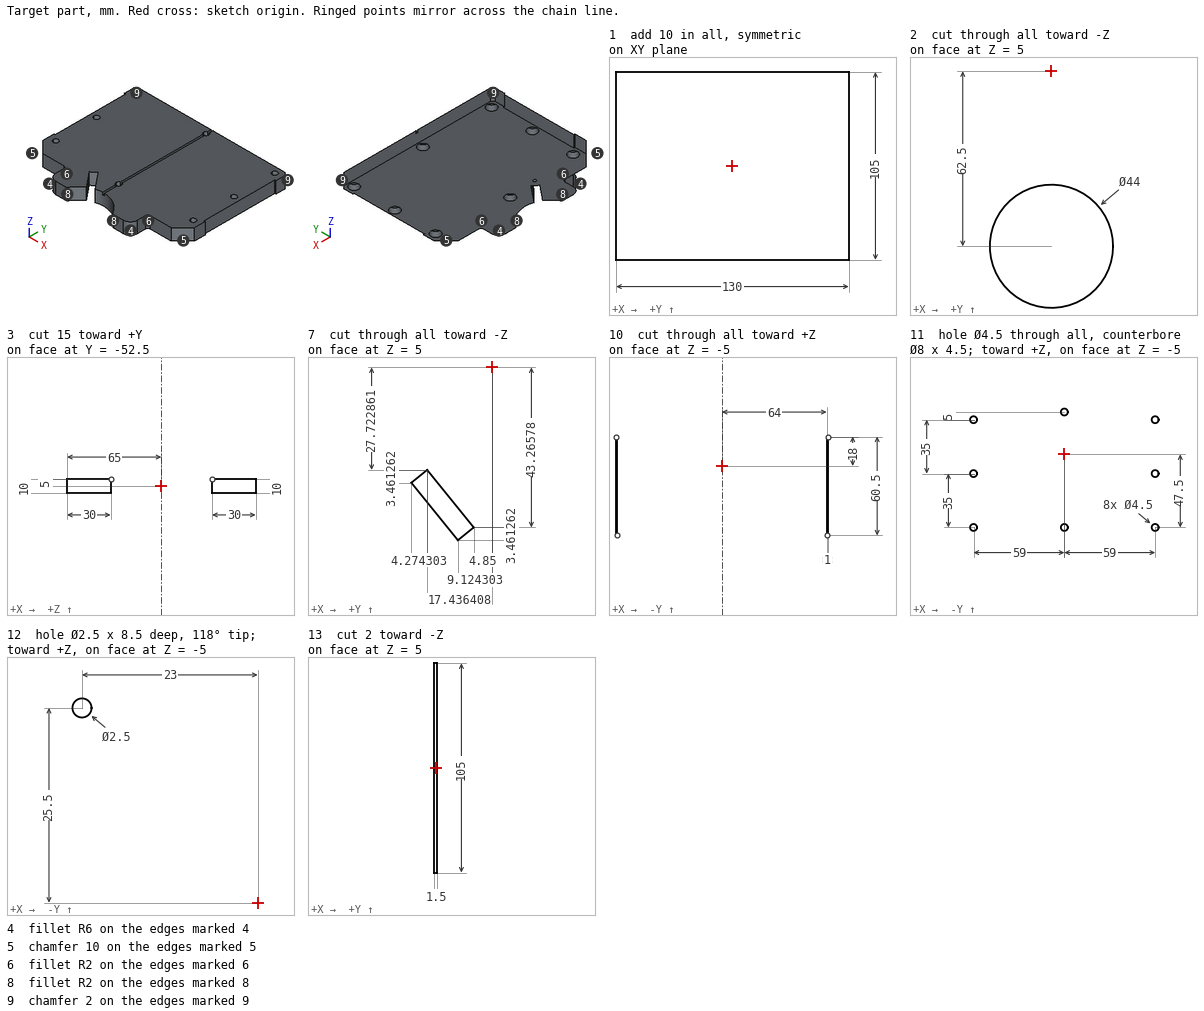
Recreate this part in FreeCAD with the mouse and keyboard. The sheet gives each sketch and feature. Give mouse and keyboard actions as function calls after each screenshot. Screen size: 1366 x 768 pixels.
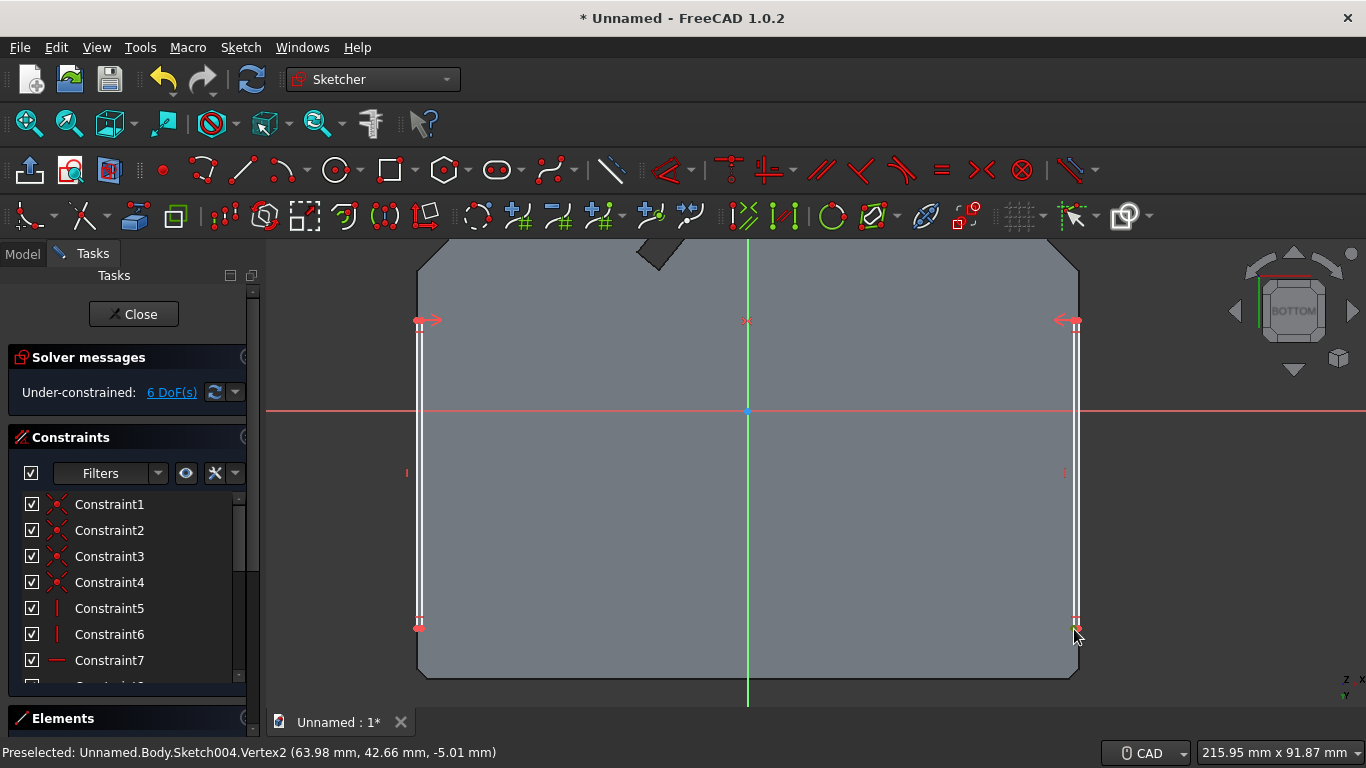
scroll(422, 629, up, 5)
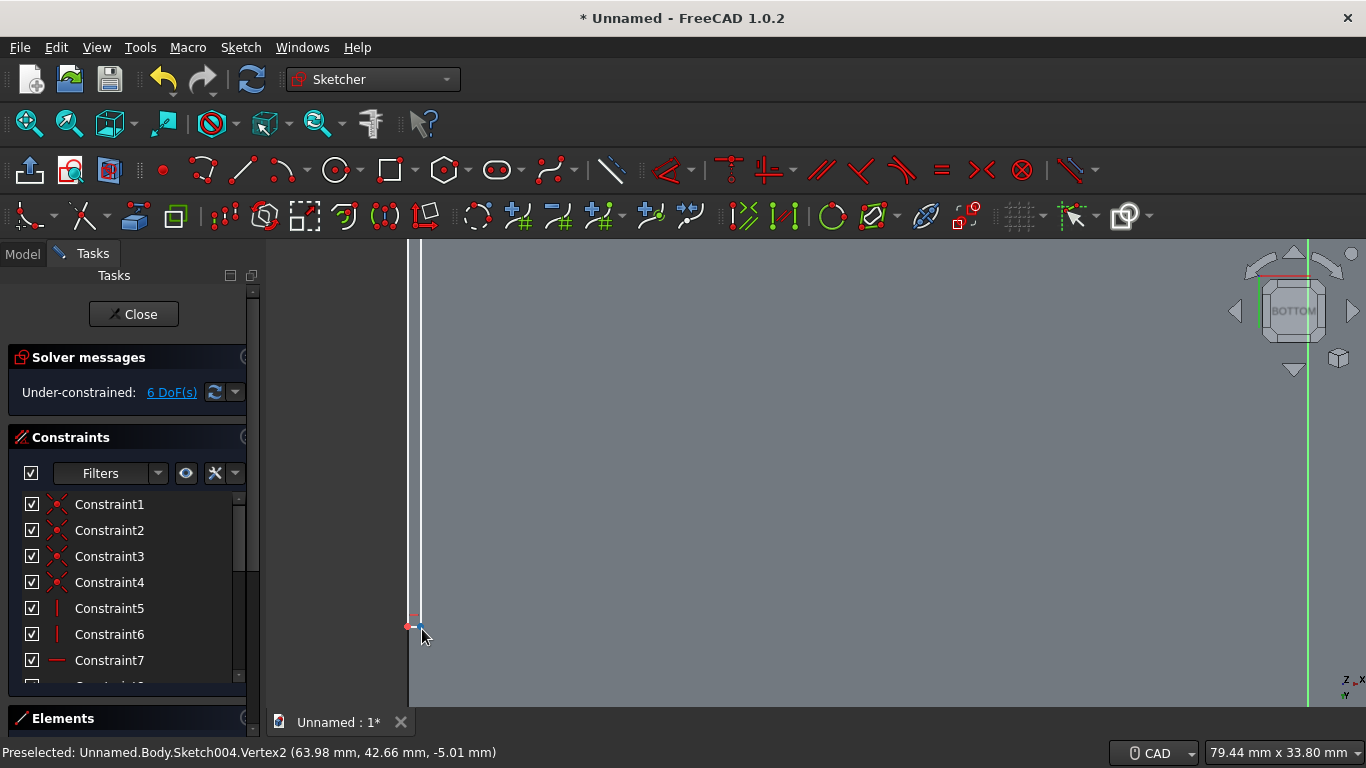
click(421, 627)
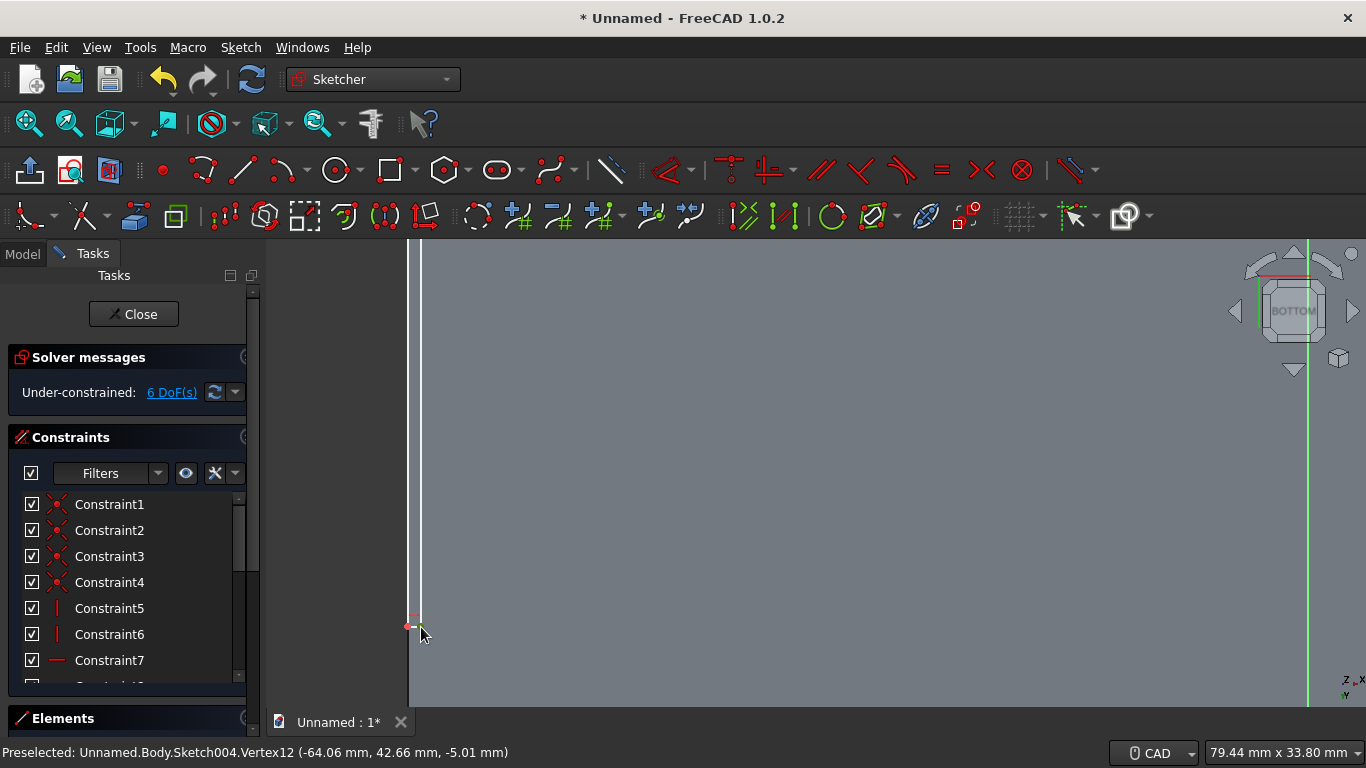
scroll(421, 629, down, 5)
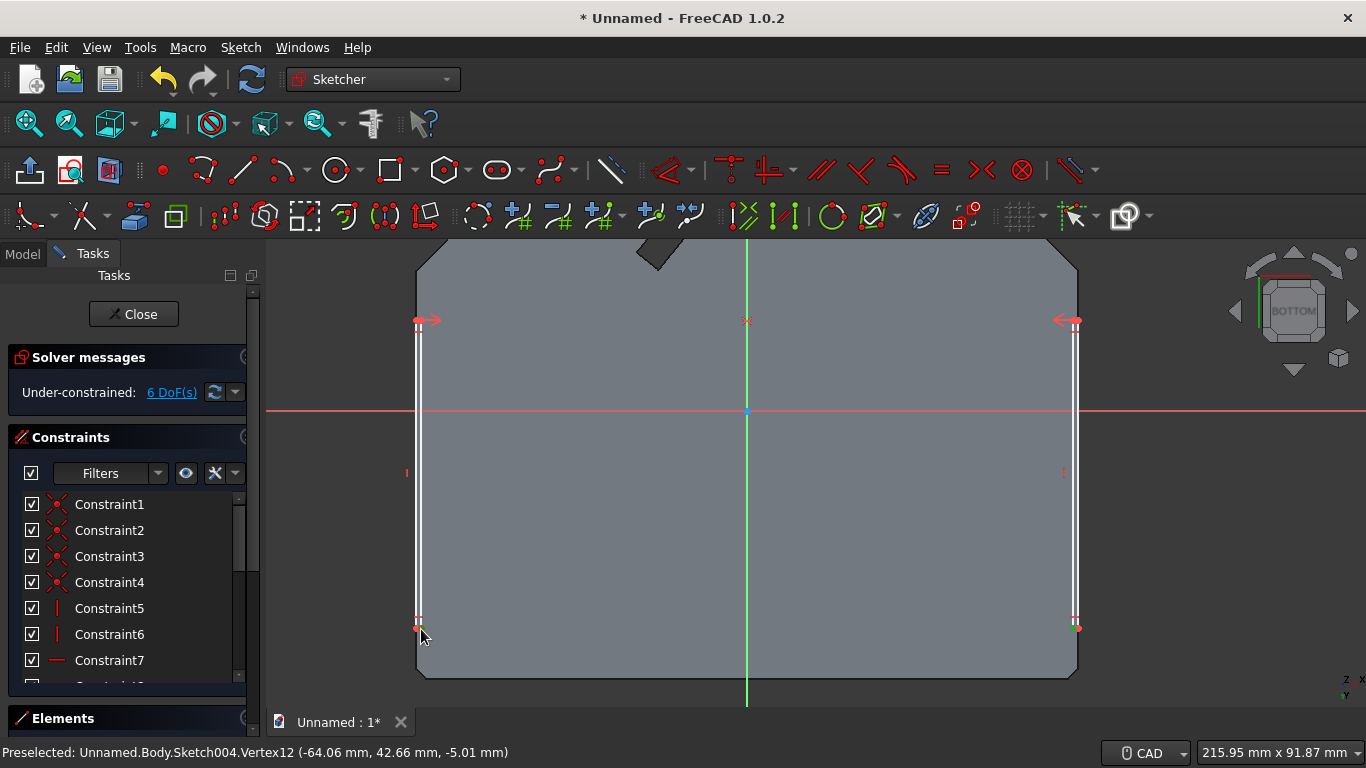
click(747, 650)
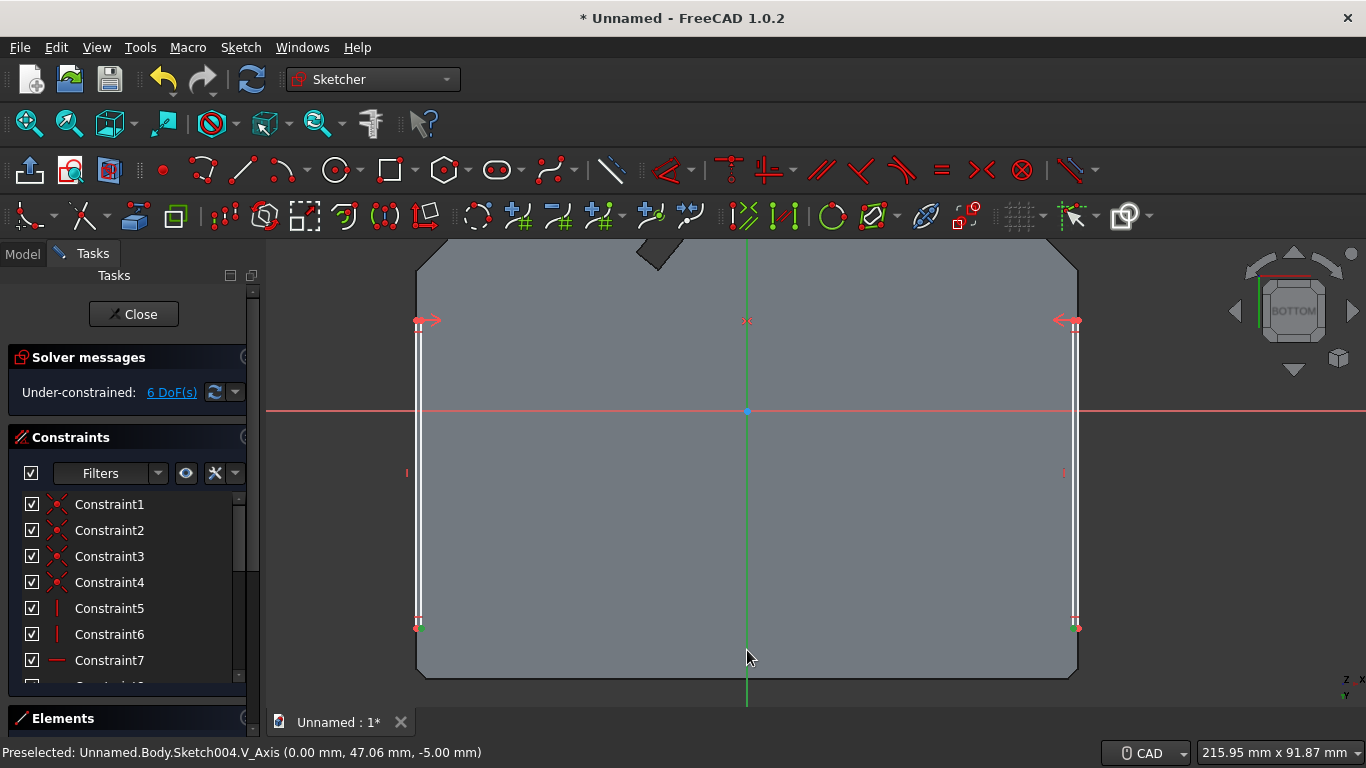
click(982, 170)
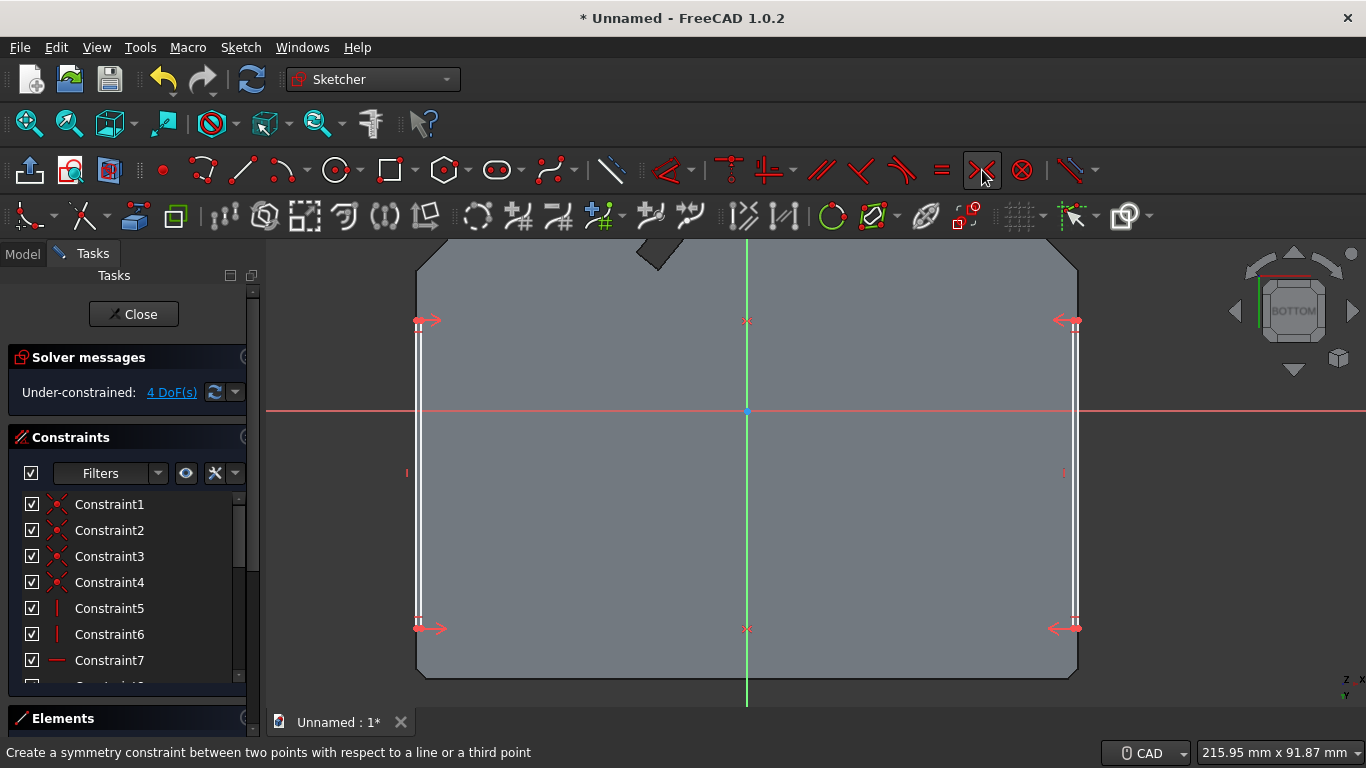
click(666, 170)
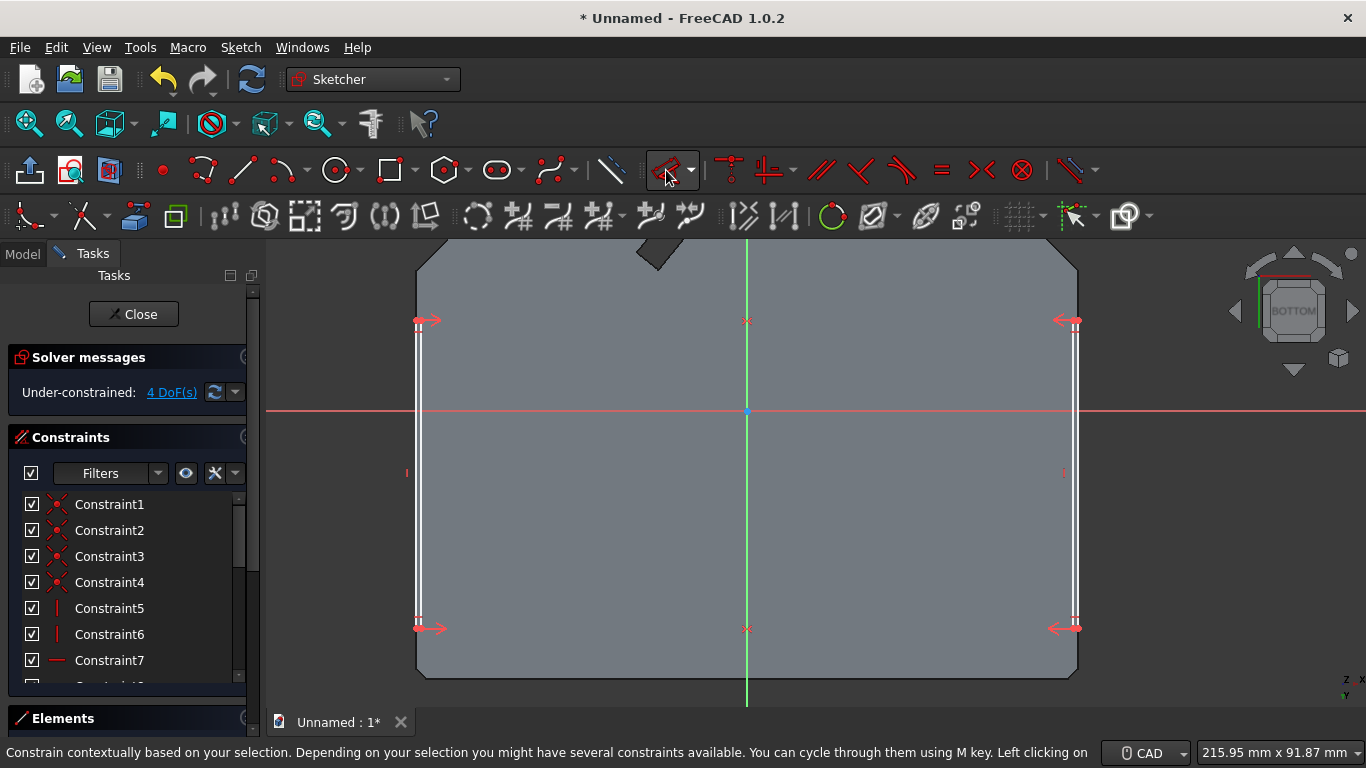
scroll(1076, 629, up, 11)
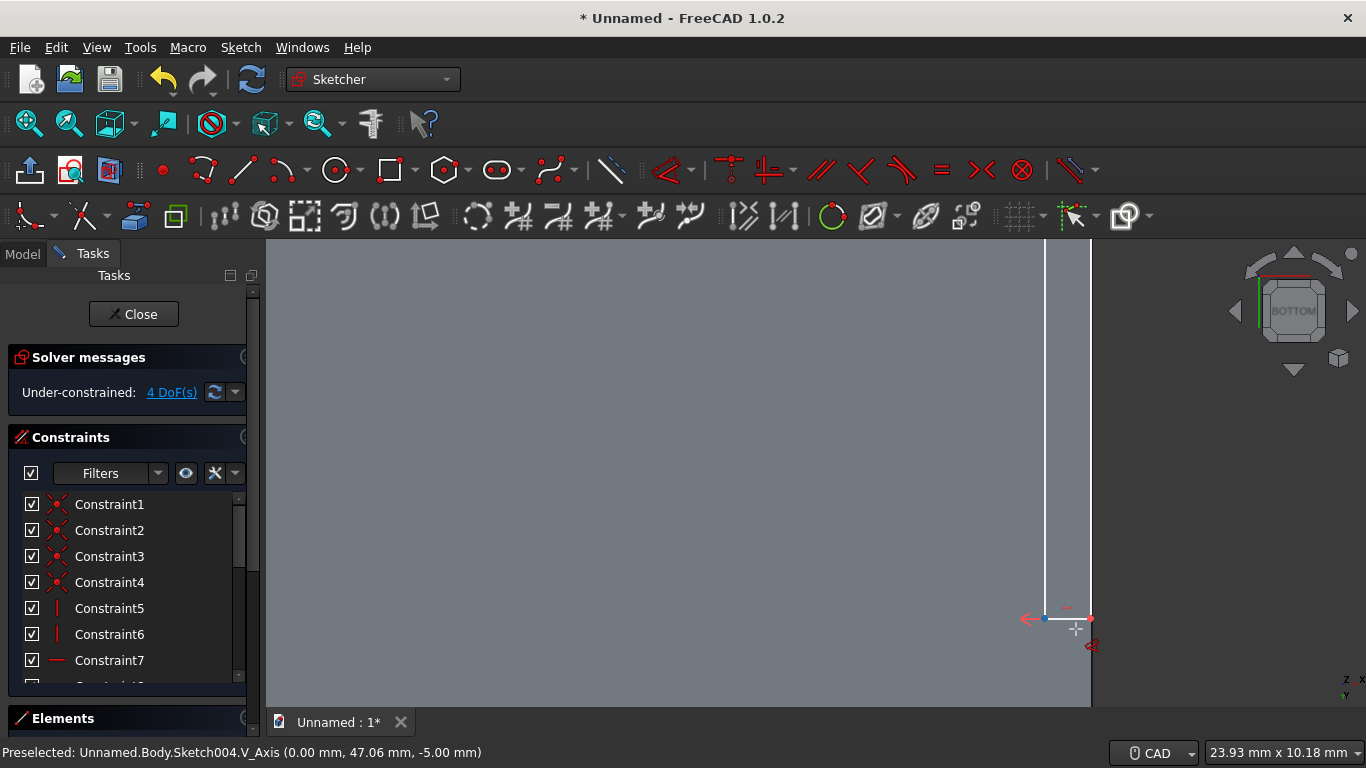
click(1068, 619)
click(1068, 653)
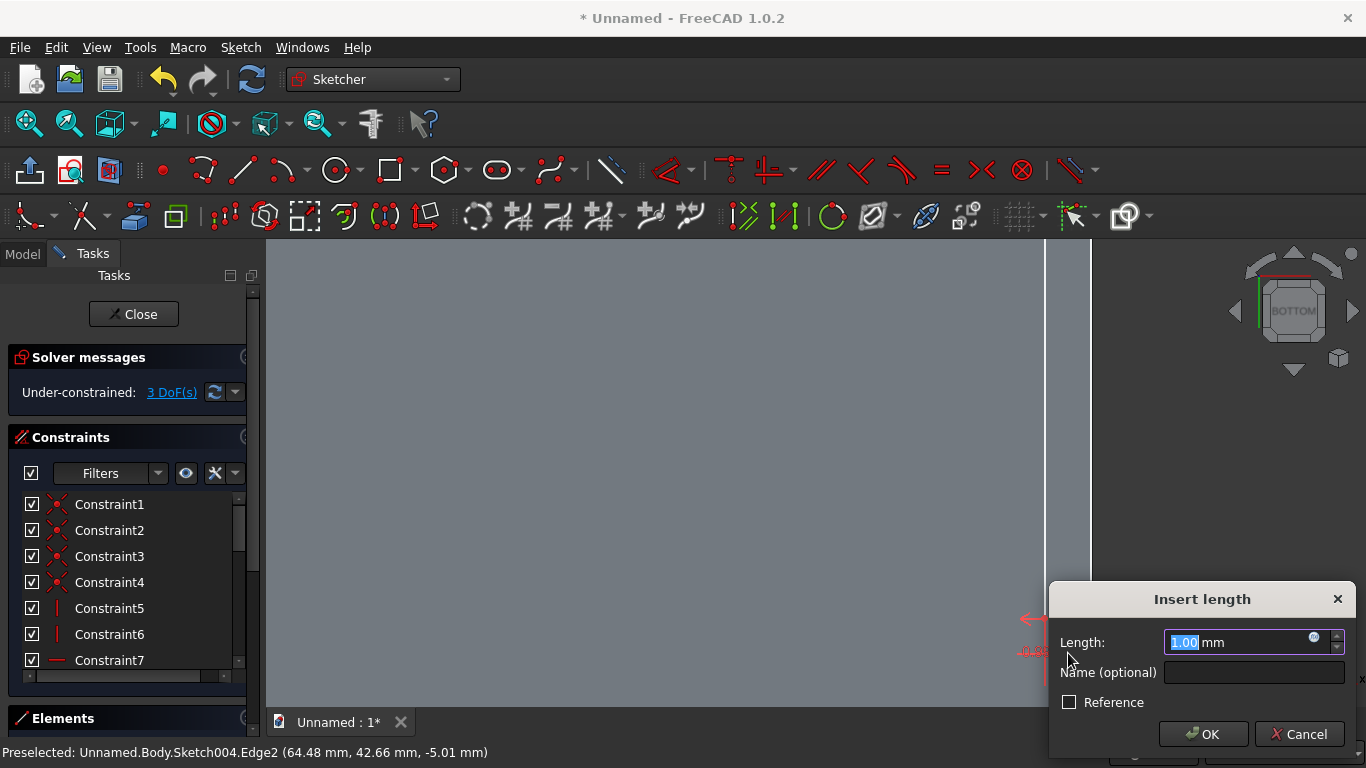
text(1)
key(Return)